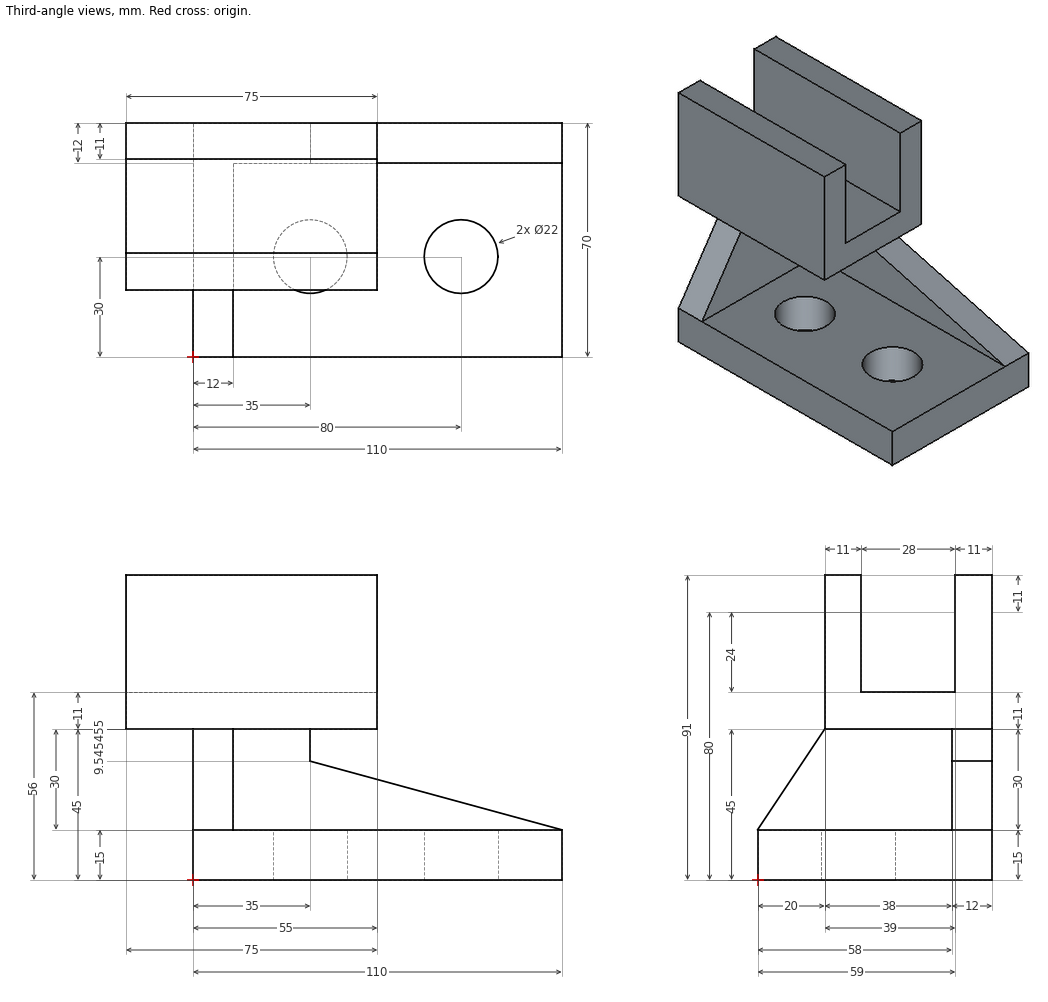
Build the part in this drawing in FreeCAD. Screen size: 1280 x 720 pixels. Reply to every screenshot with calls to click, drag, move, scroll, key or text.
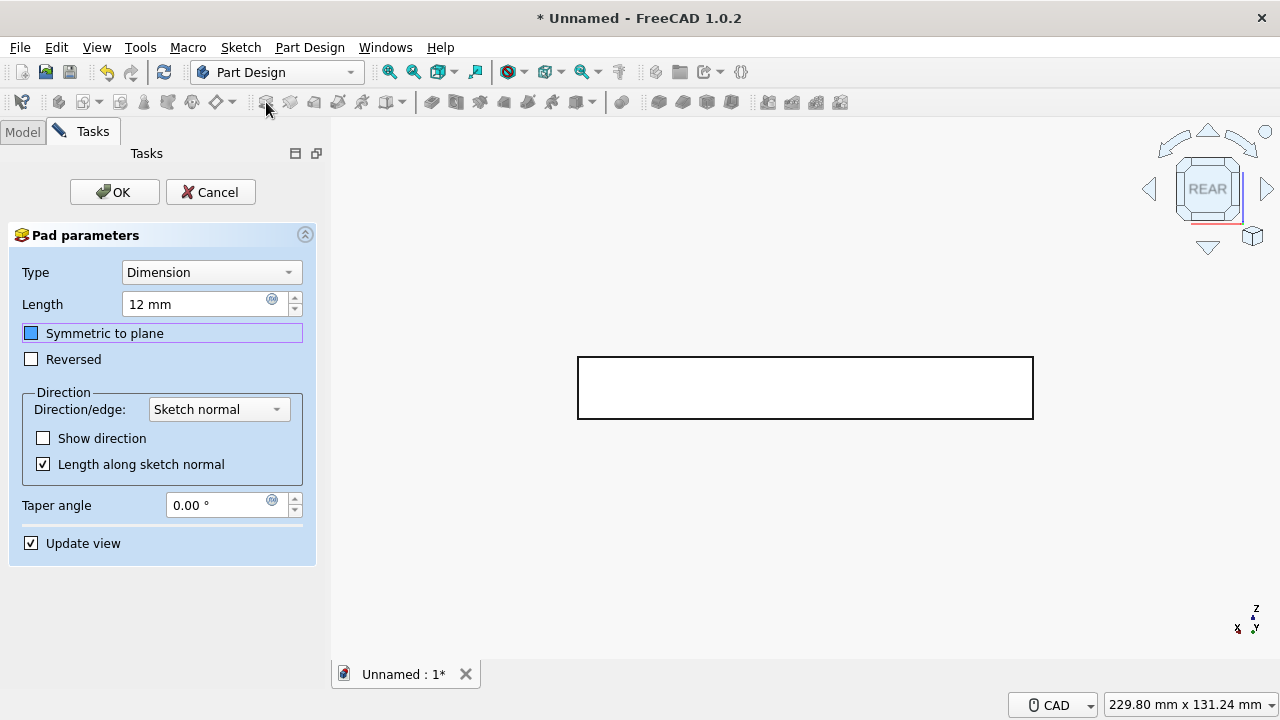
click(30, 359)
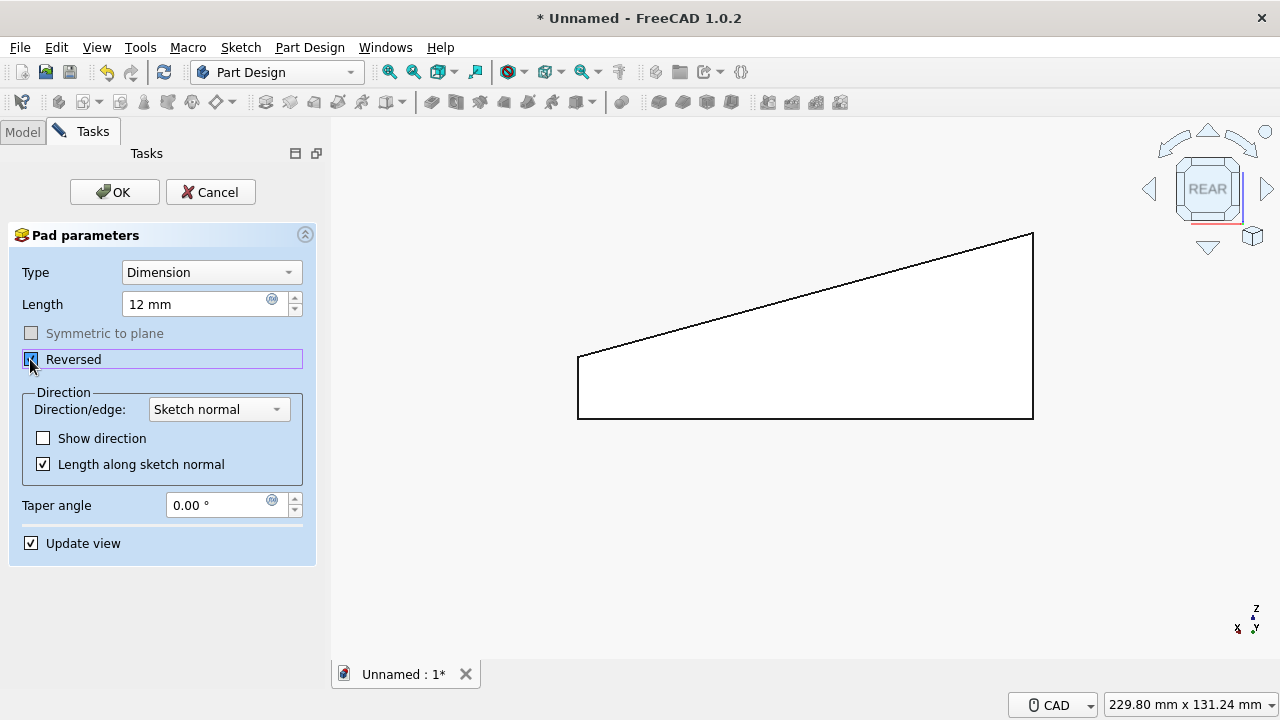
click(115, 192)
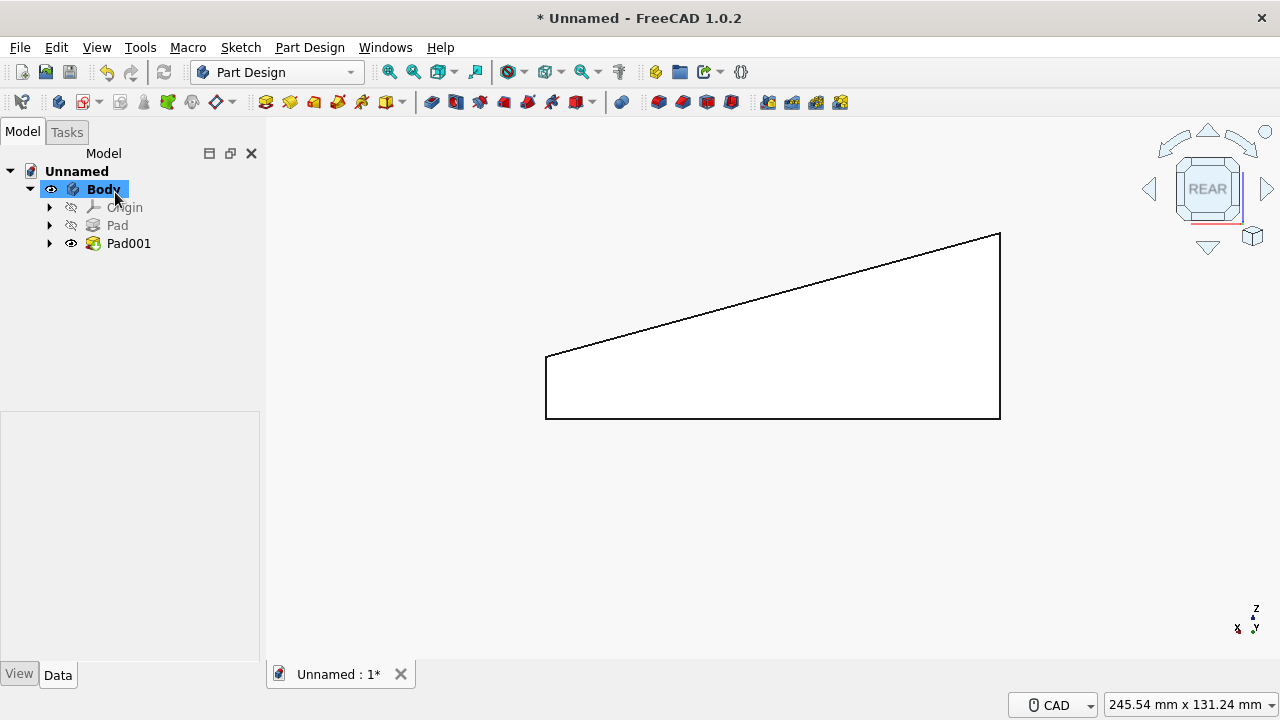
key(v)
key(f)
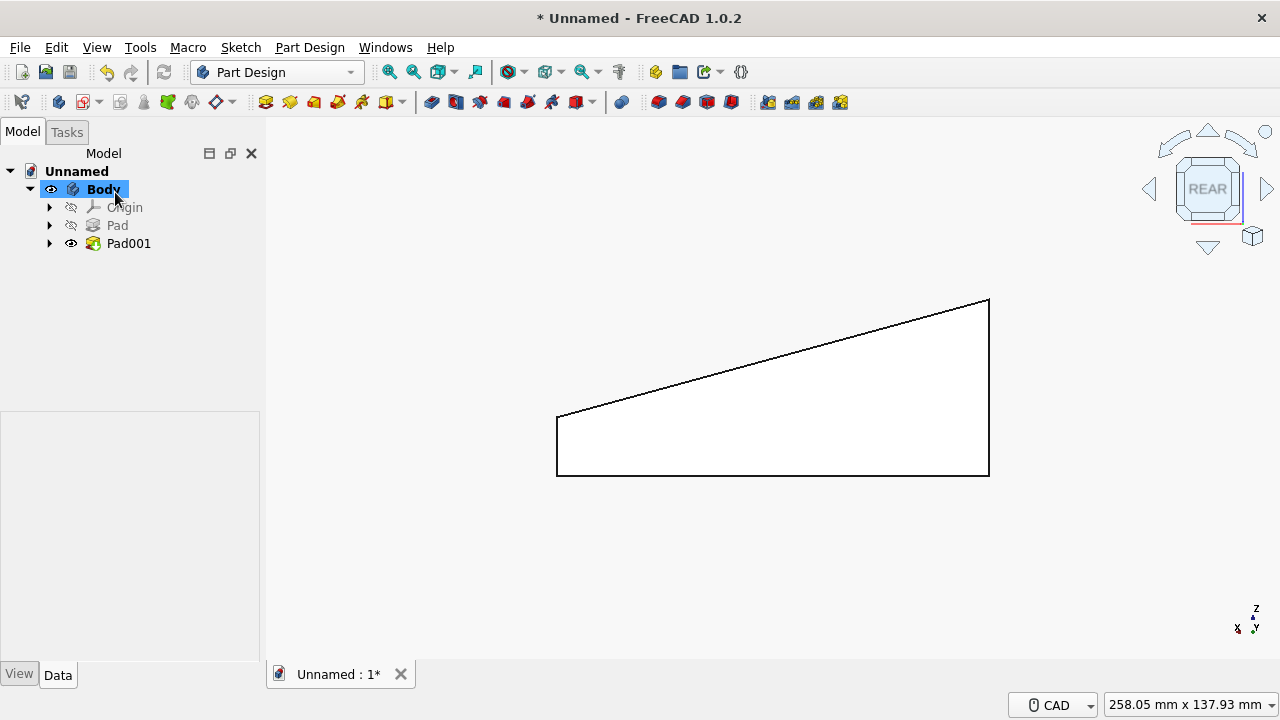
key(6)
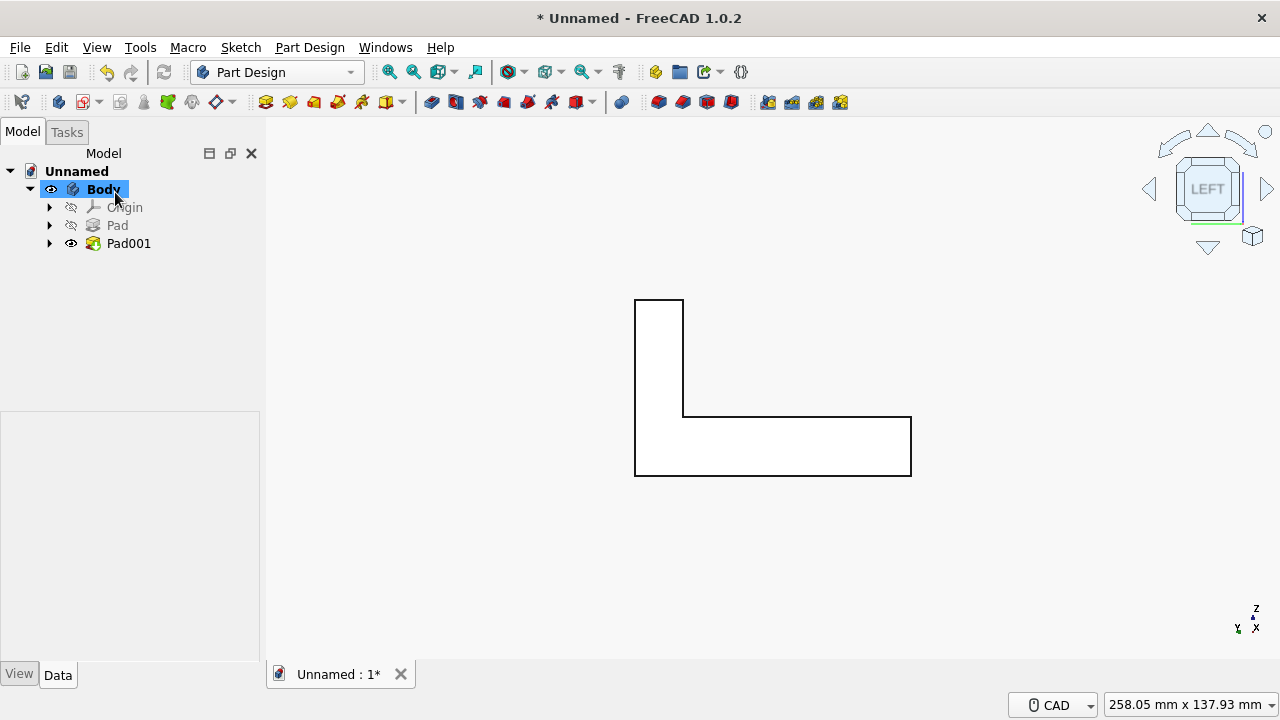
click(390, 72)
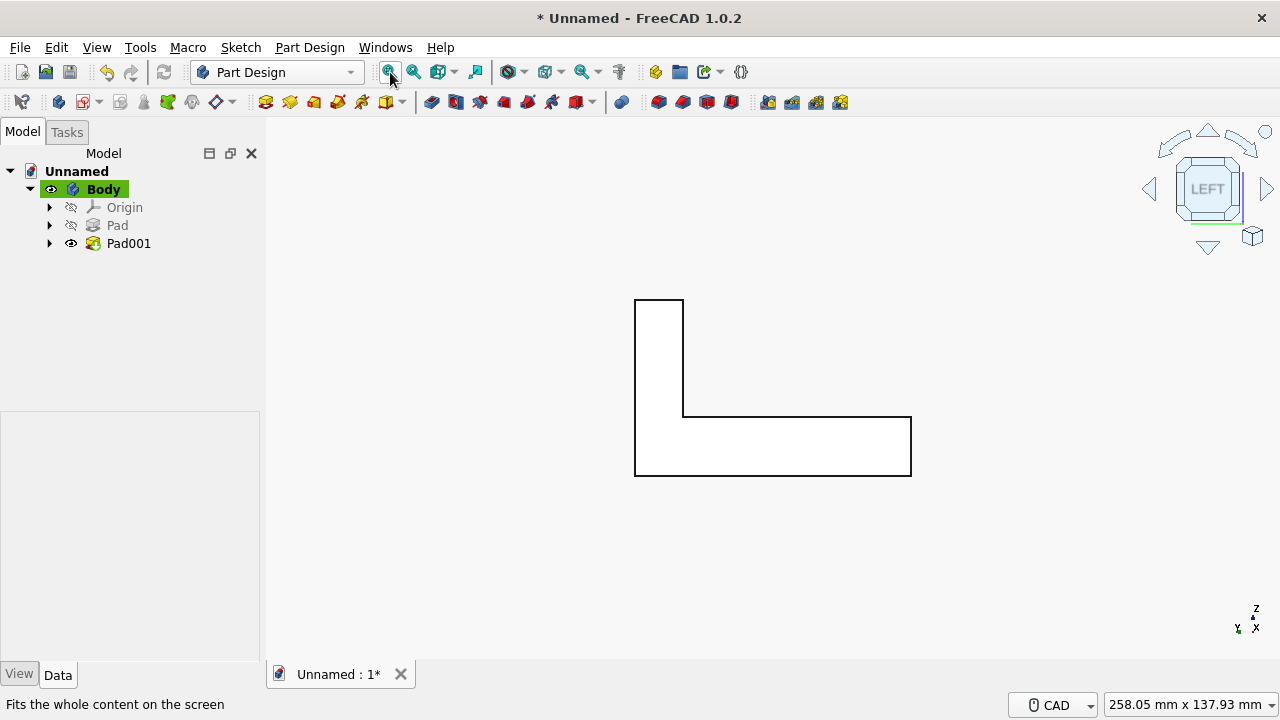
click(694, 438)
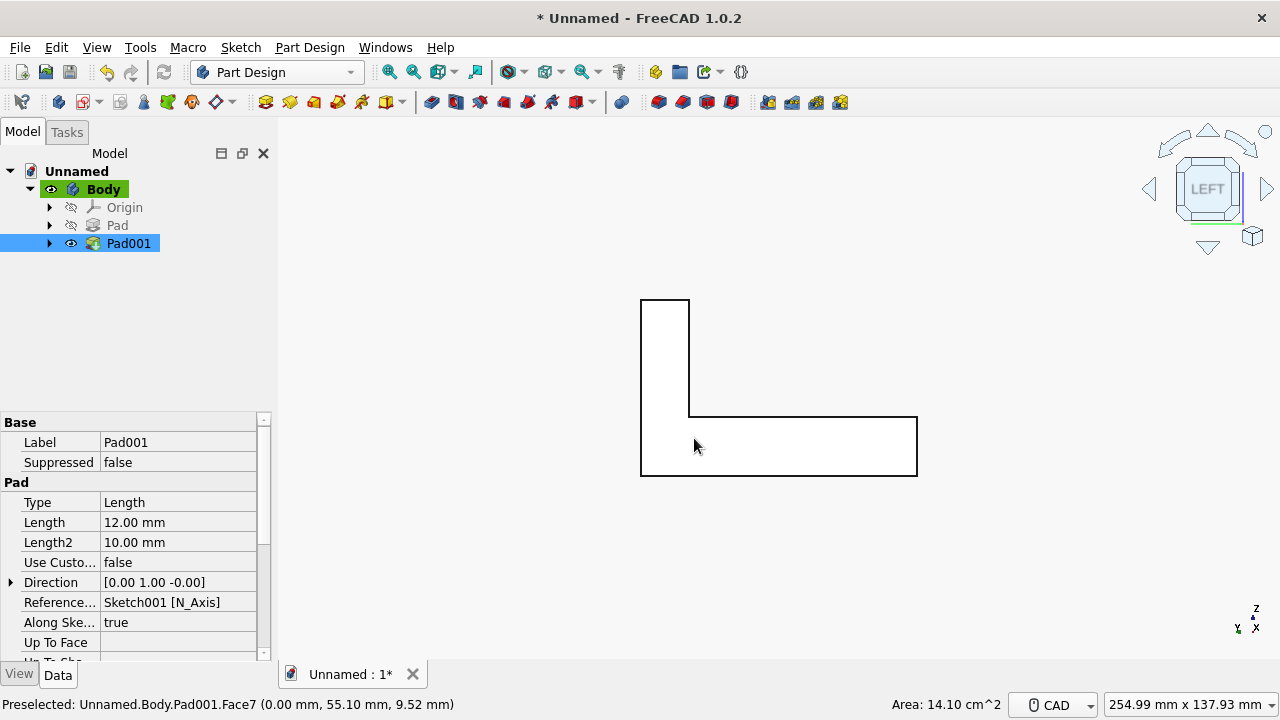
click(84, 102)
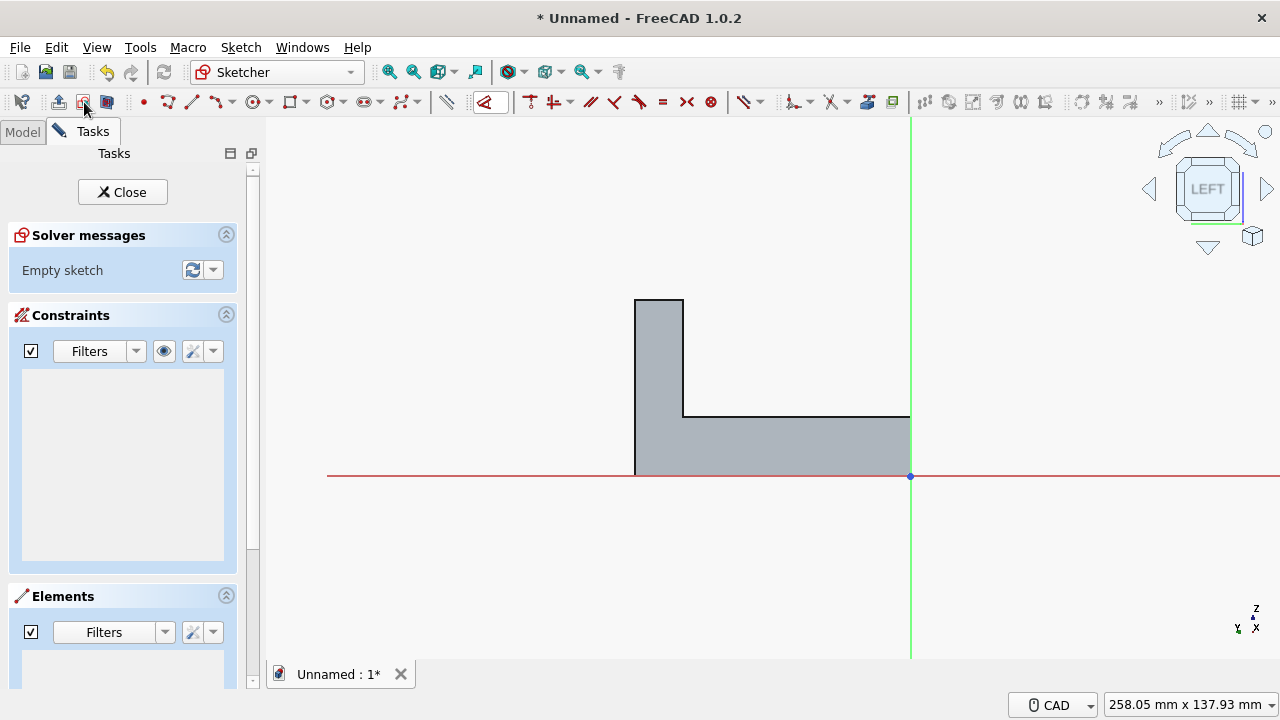
scroll(909, 388, up, 3)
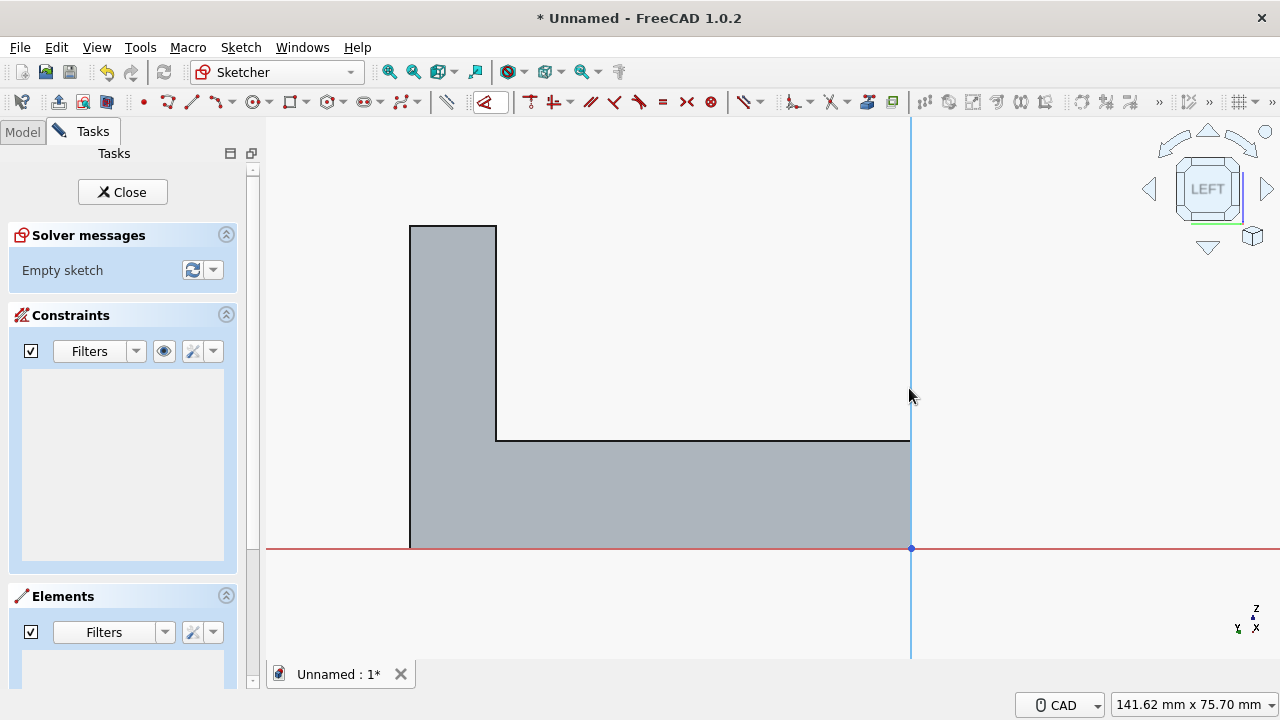
click(168, 102)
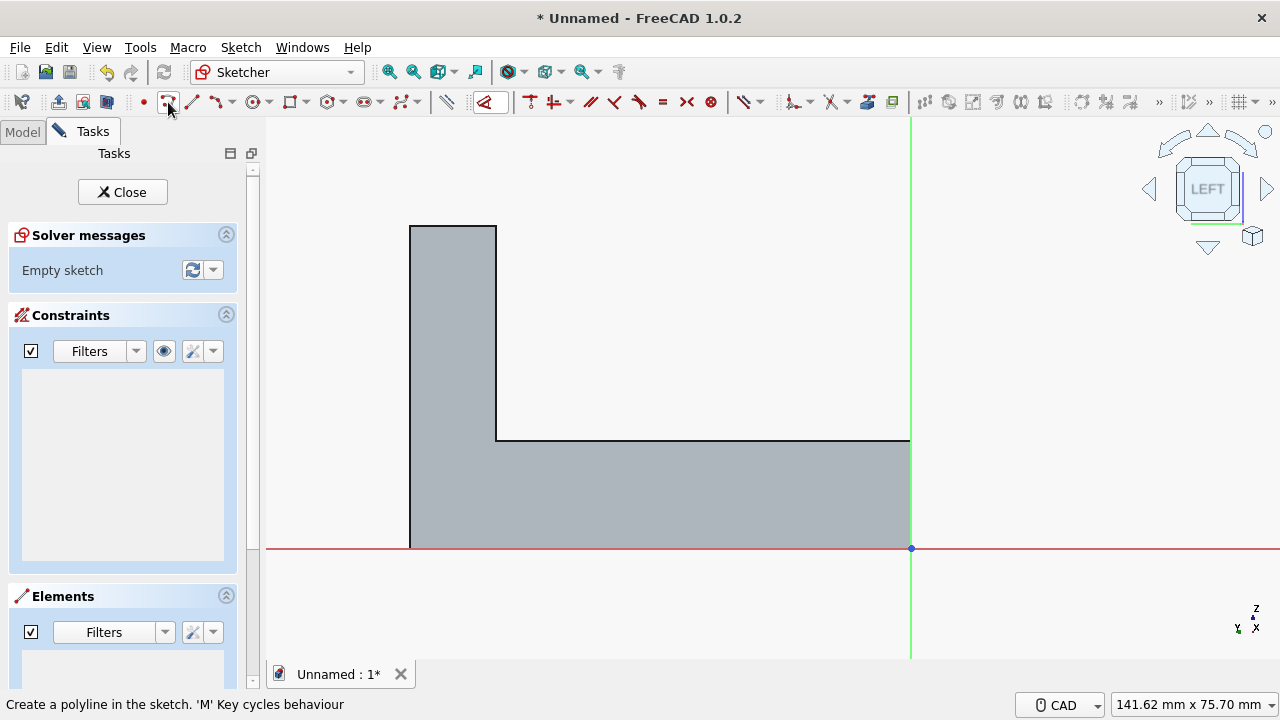
click(911, 441)
click(768, 226)
click(496, 226)
click(496, 441)
click(911, 442)
key(Escape)
key(Escape)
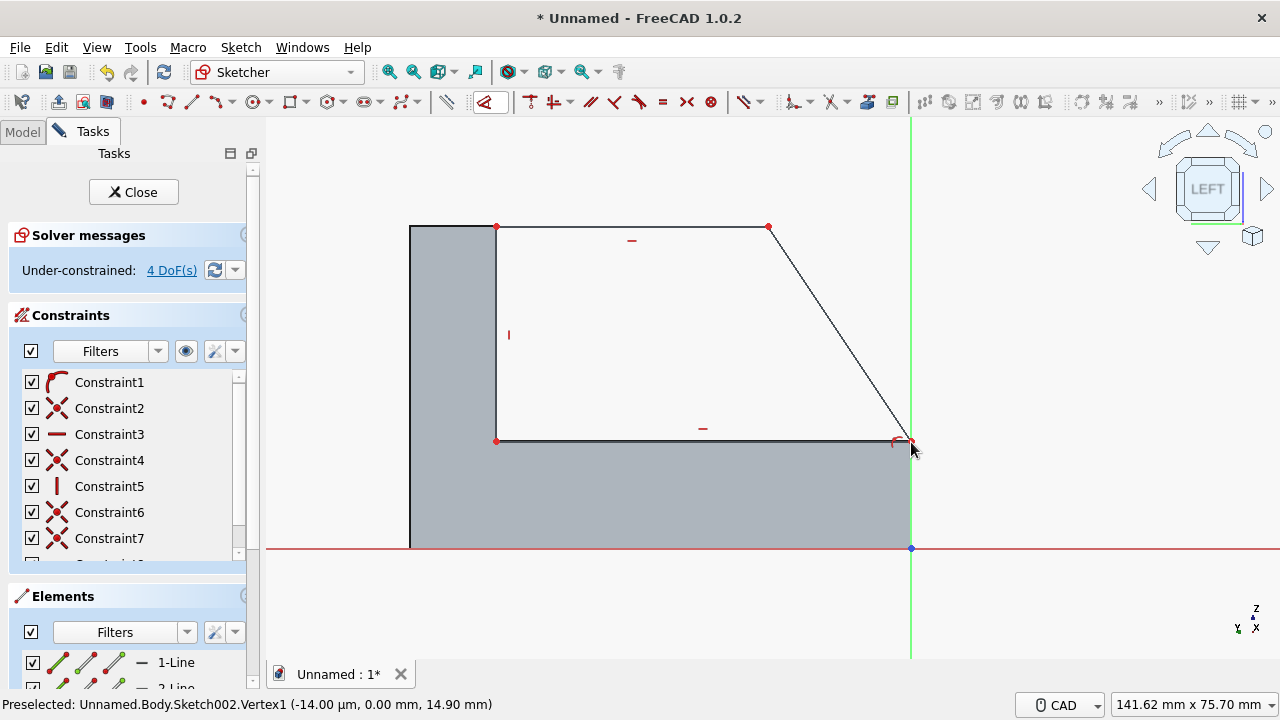
click(686, 227)